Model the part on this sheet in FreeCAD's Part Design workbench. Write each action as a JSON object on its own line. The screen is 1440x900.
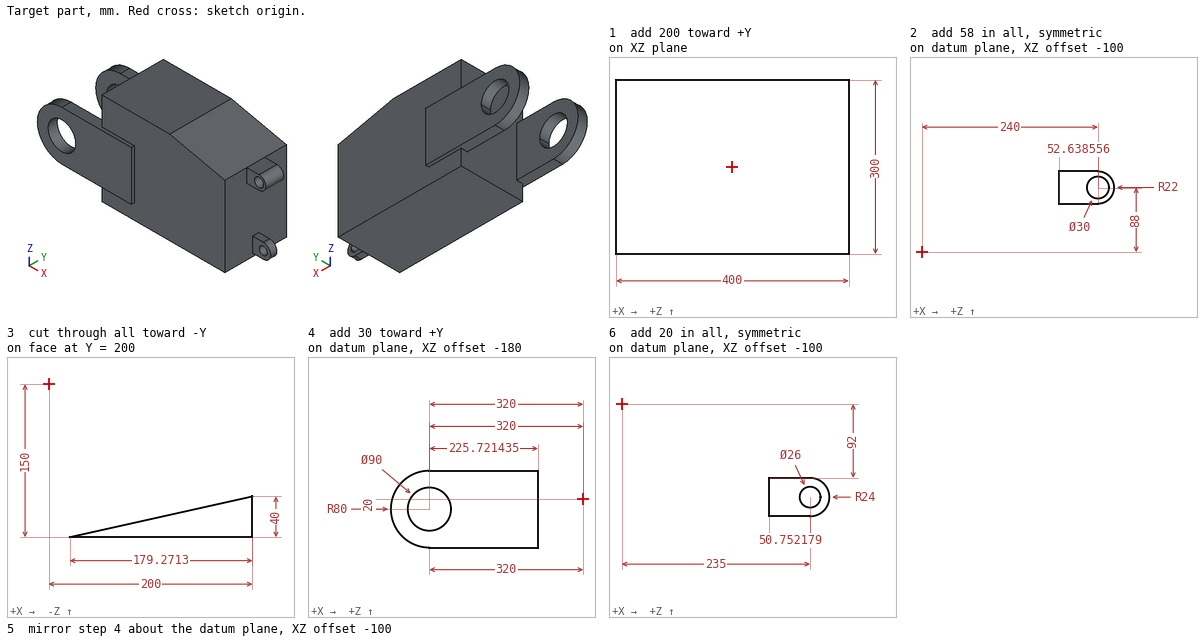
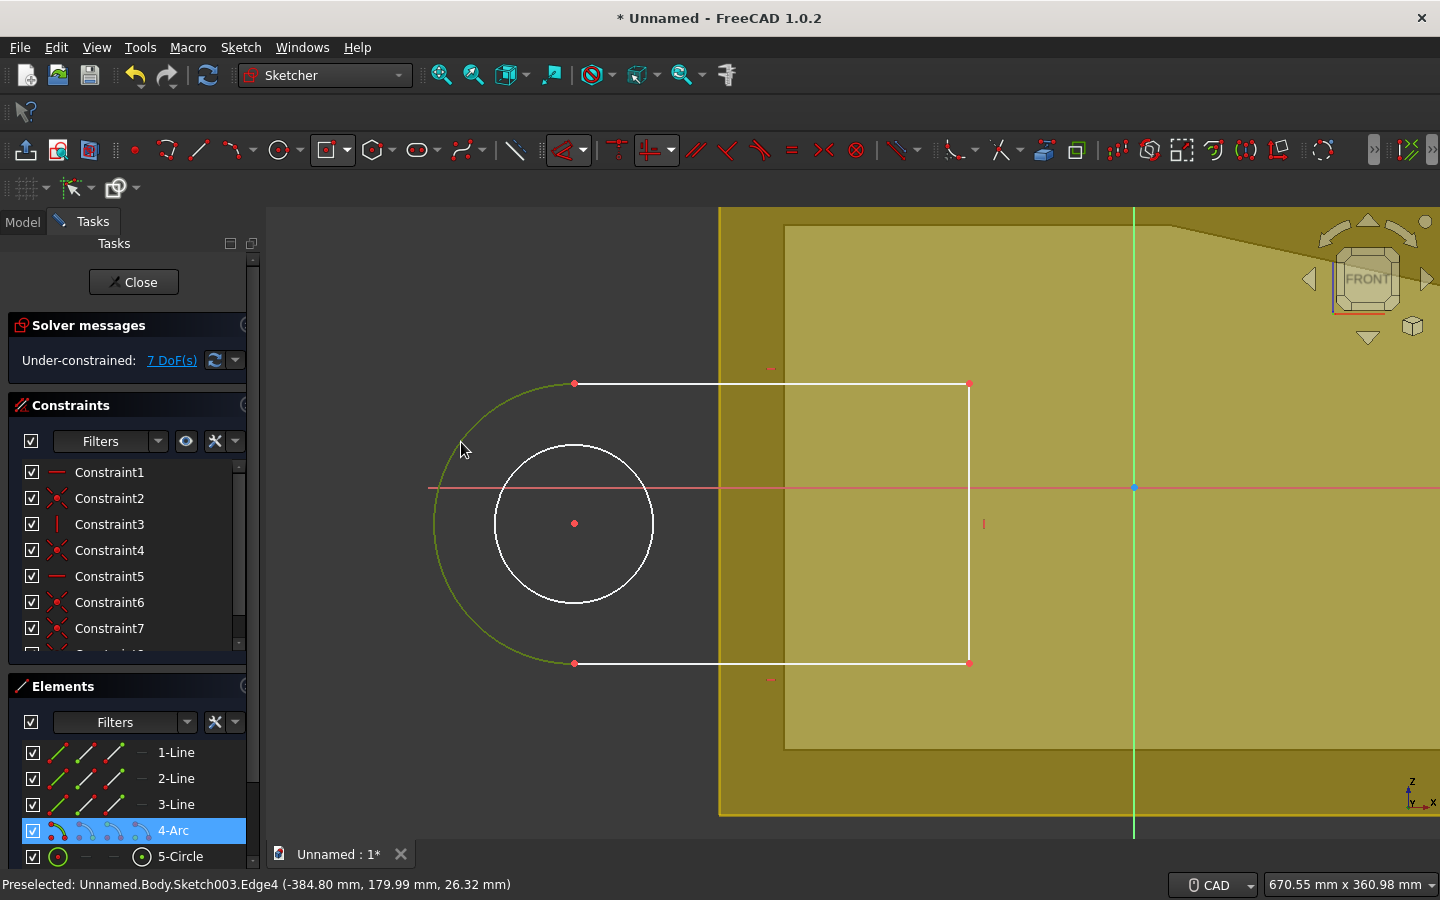
{"action": "left_click", "coordinate": [586, 150]}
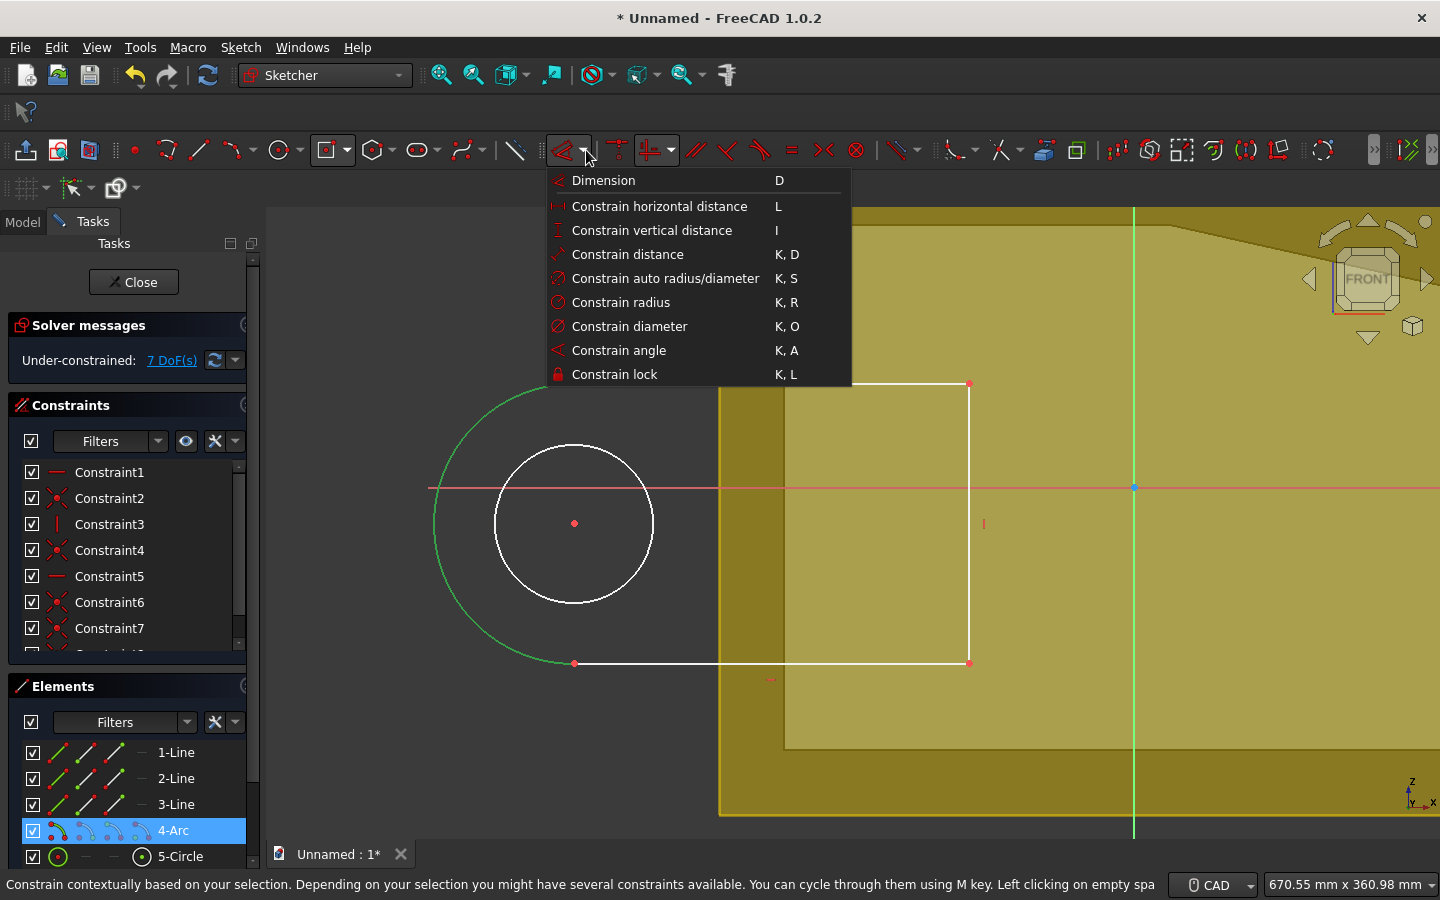
{"action": "left_click", "coordinate": [699, 302]}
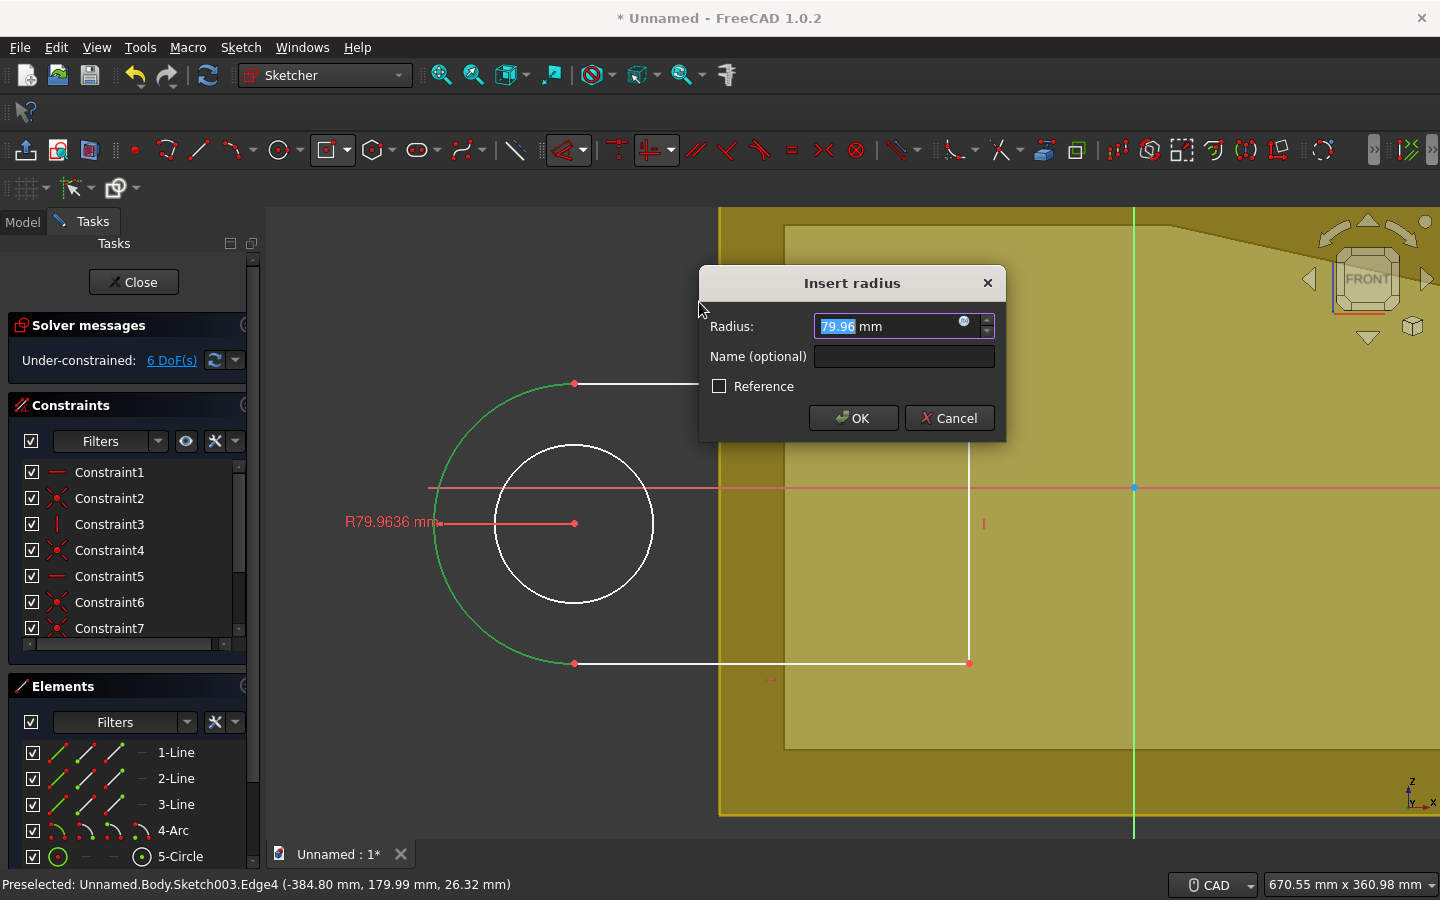
{"action": "type", "text": "80"}
{"action": "key", "text": "Return"}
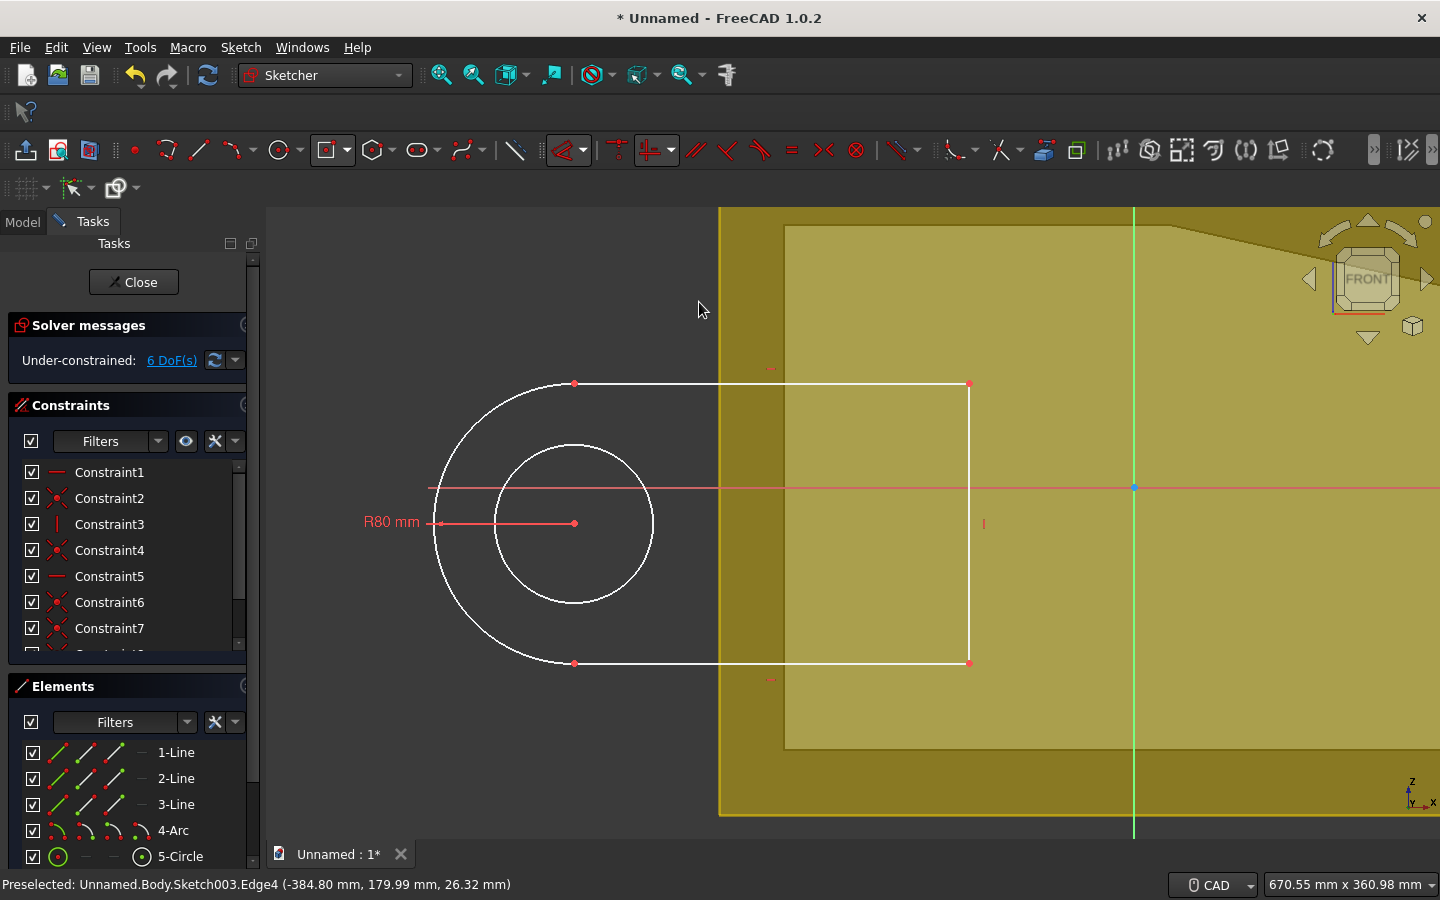
{"action": "left_click", "coordinate": [630, 468]}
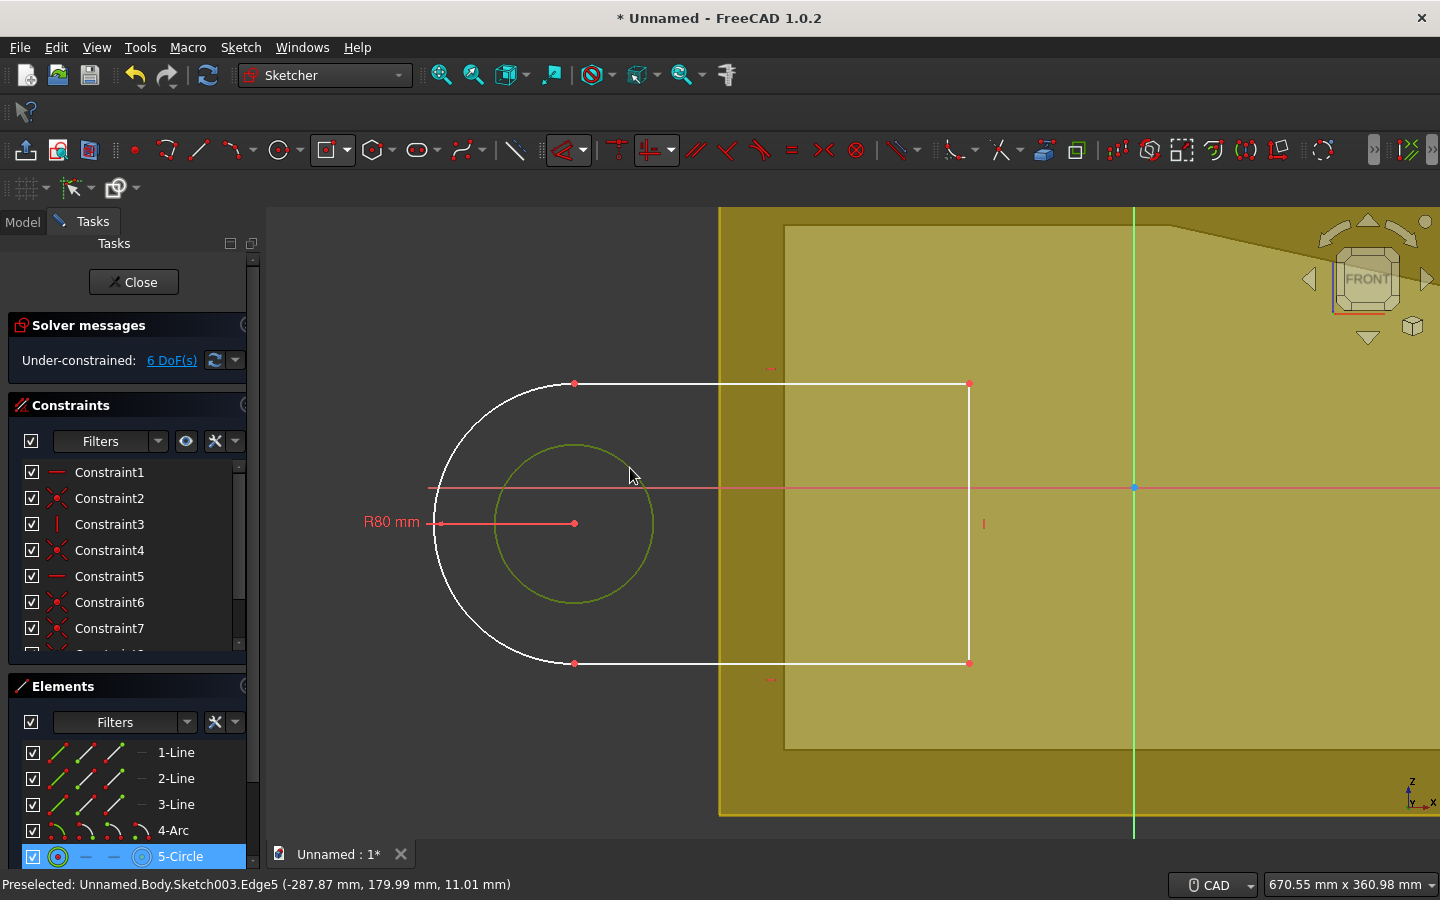
{"action": "left_click", "coordinate": [586, 150]}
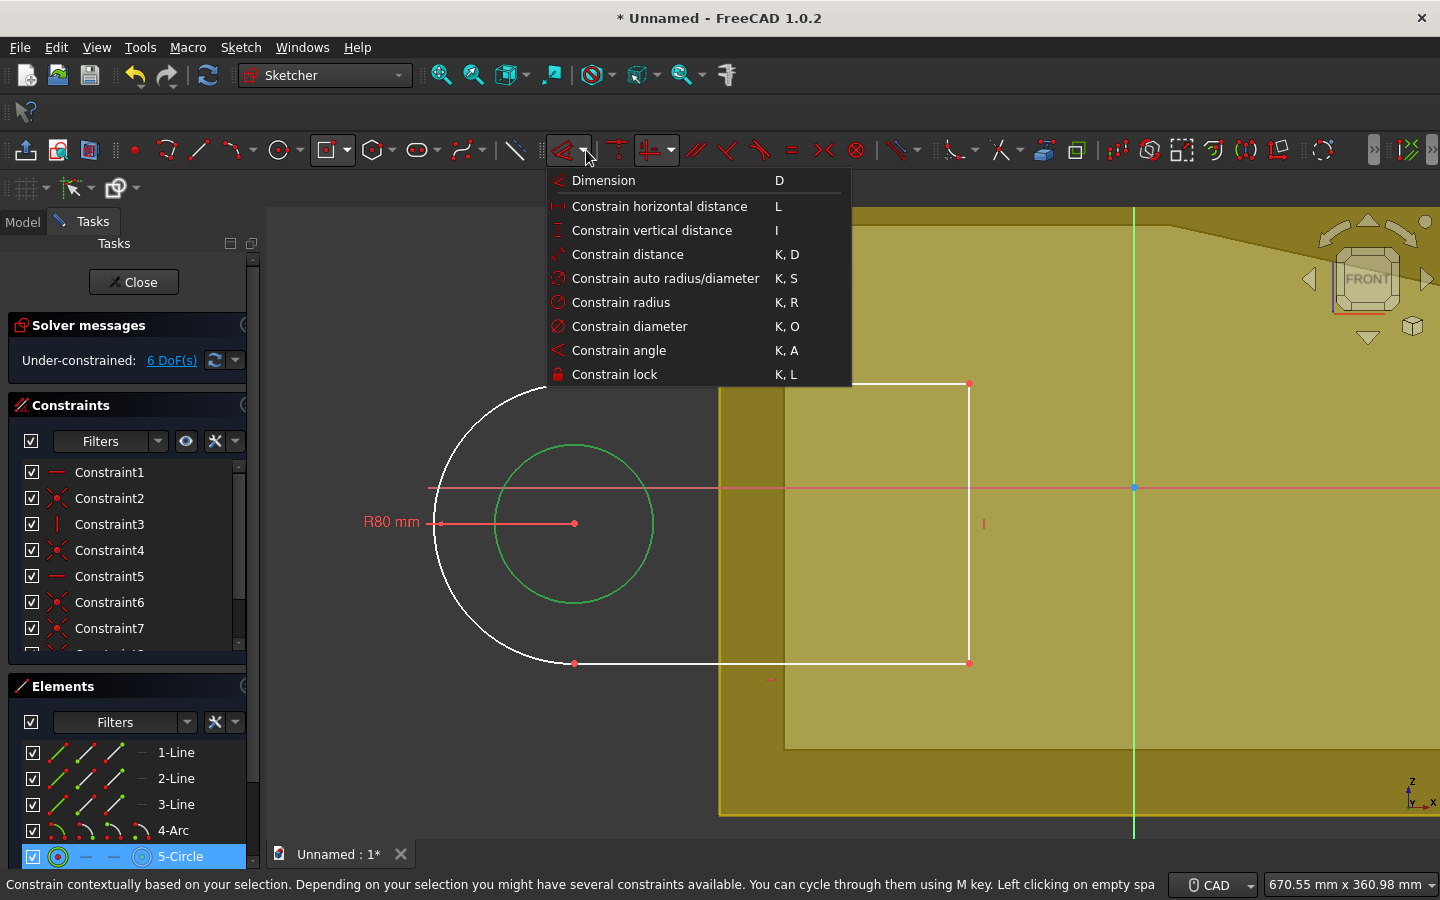
{"action": "left_click", "coordinate": [699, 326]}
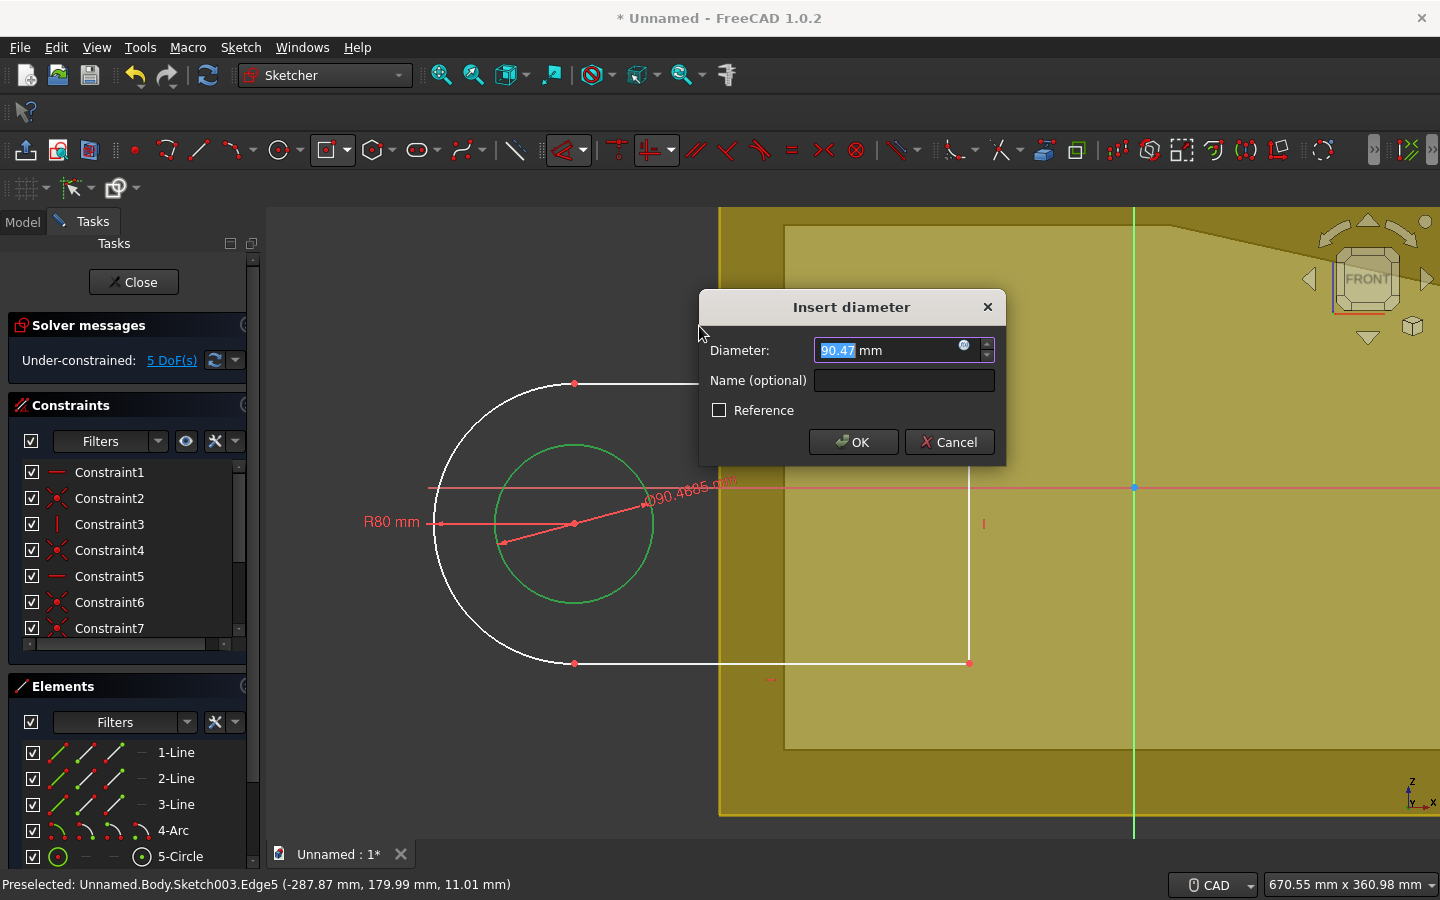
{"action": "type", "text": "90"}
{"action": "key", "text": "Return"}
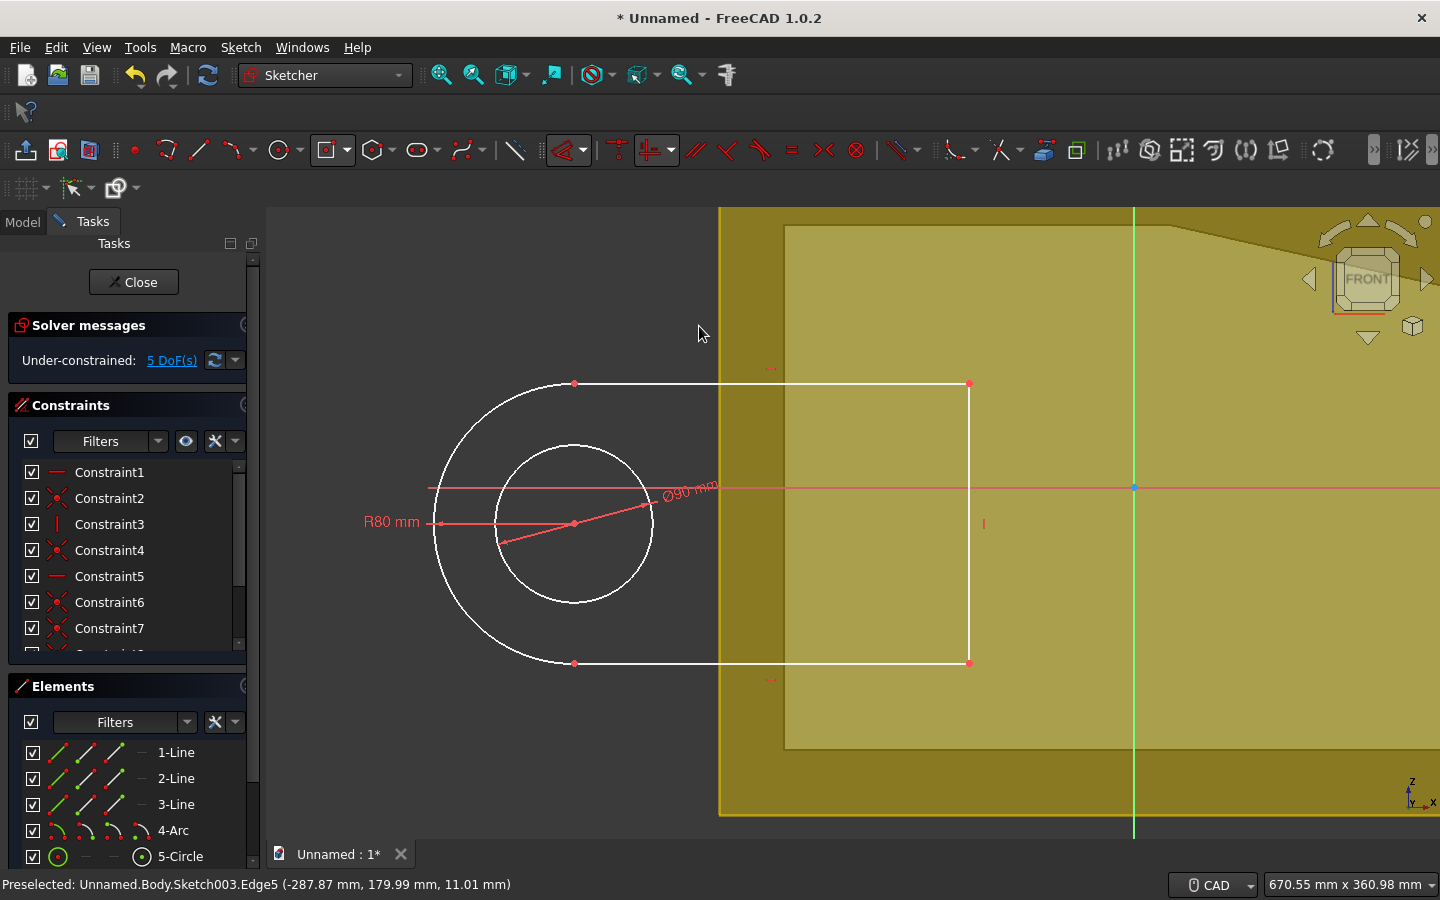
{"action": "left_click", "coordinate": [574, 524]}